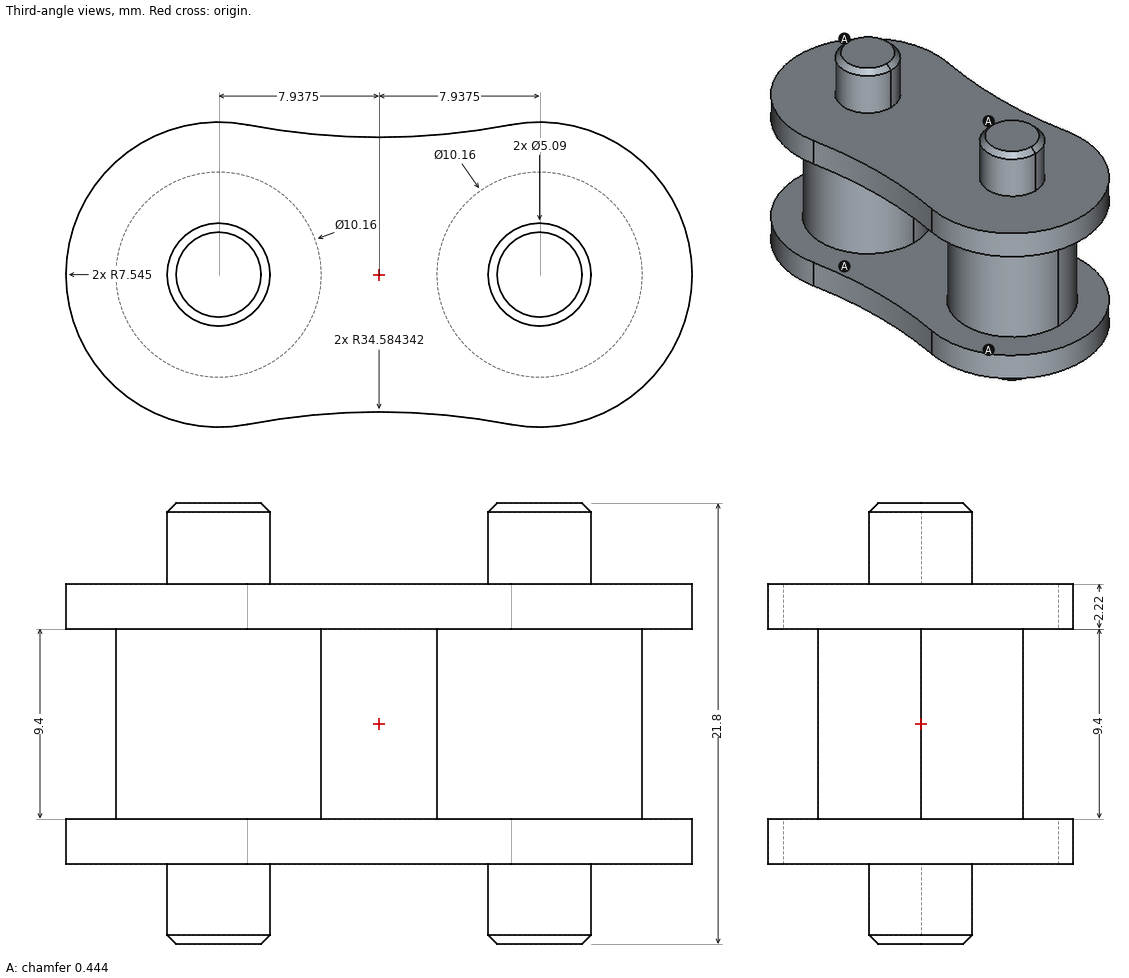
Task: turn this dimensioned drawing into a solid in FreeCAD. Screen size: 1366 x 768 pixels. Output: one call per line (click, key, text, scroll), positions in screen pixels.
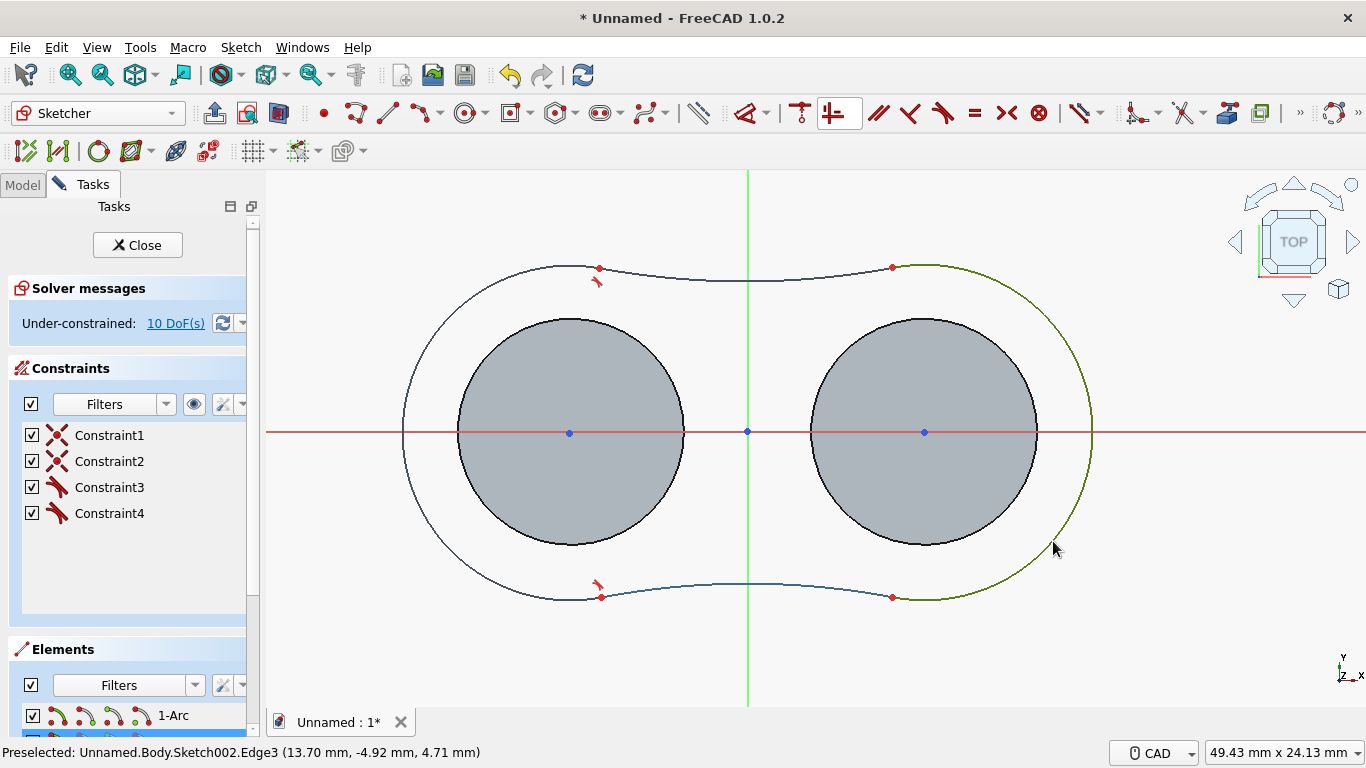
key(t)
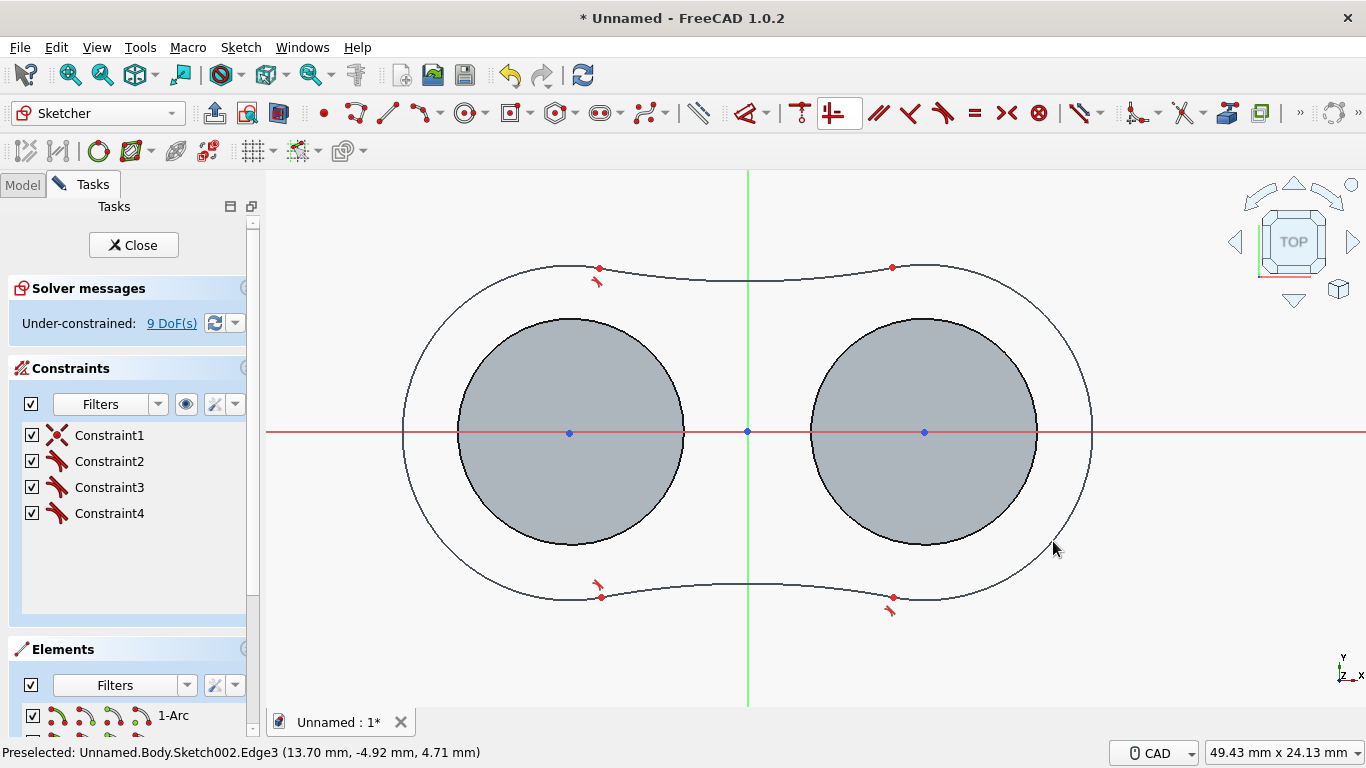
click(1053, 541)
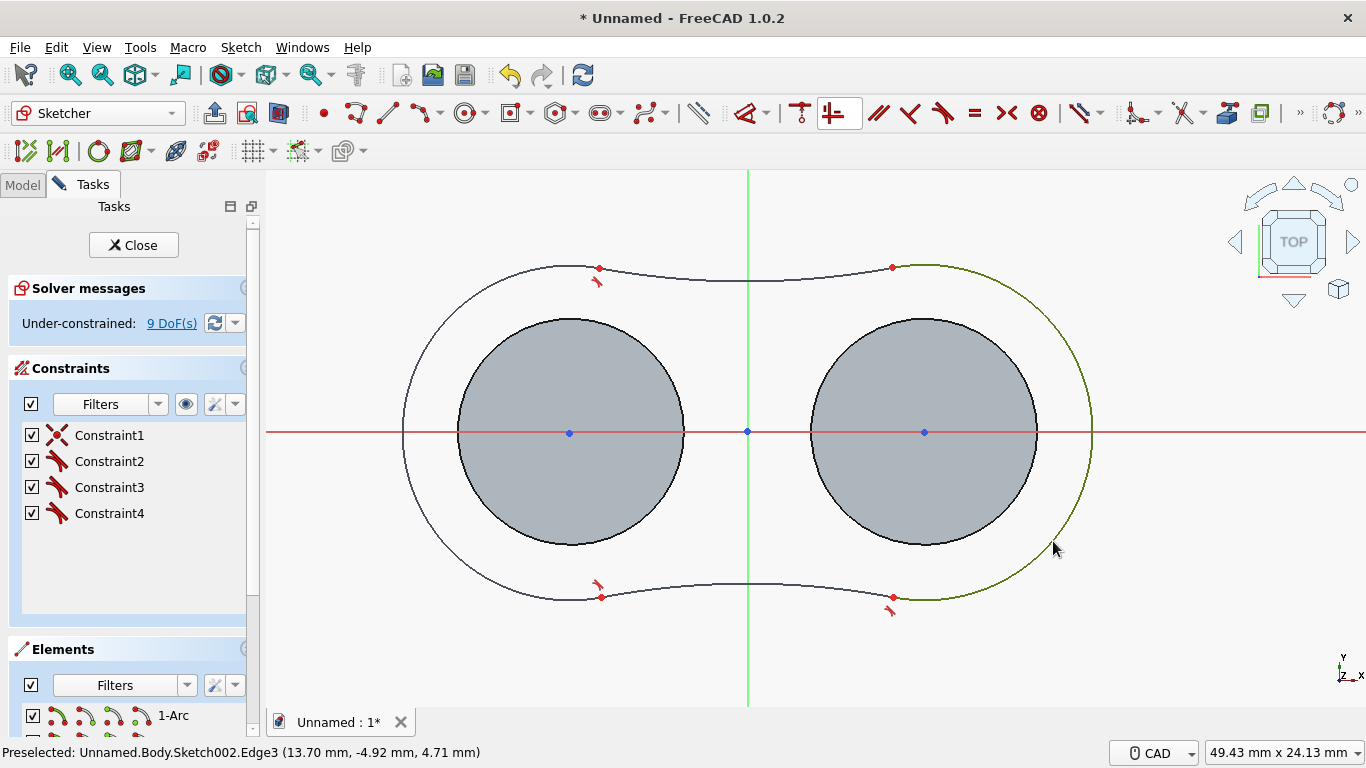
click(687, 279)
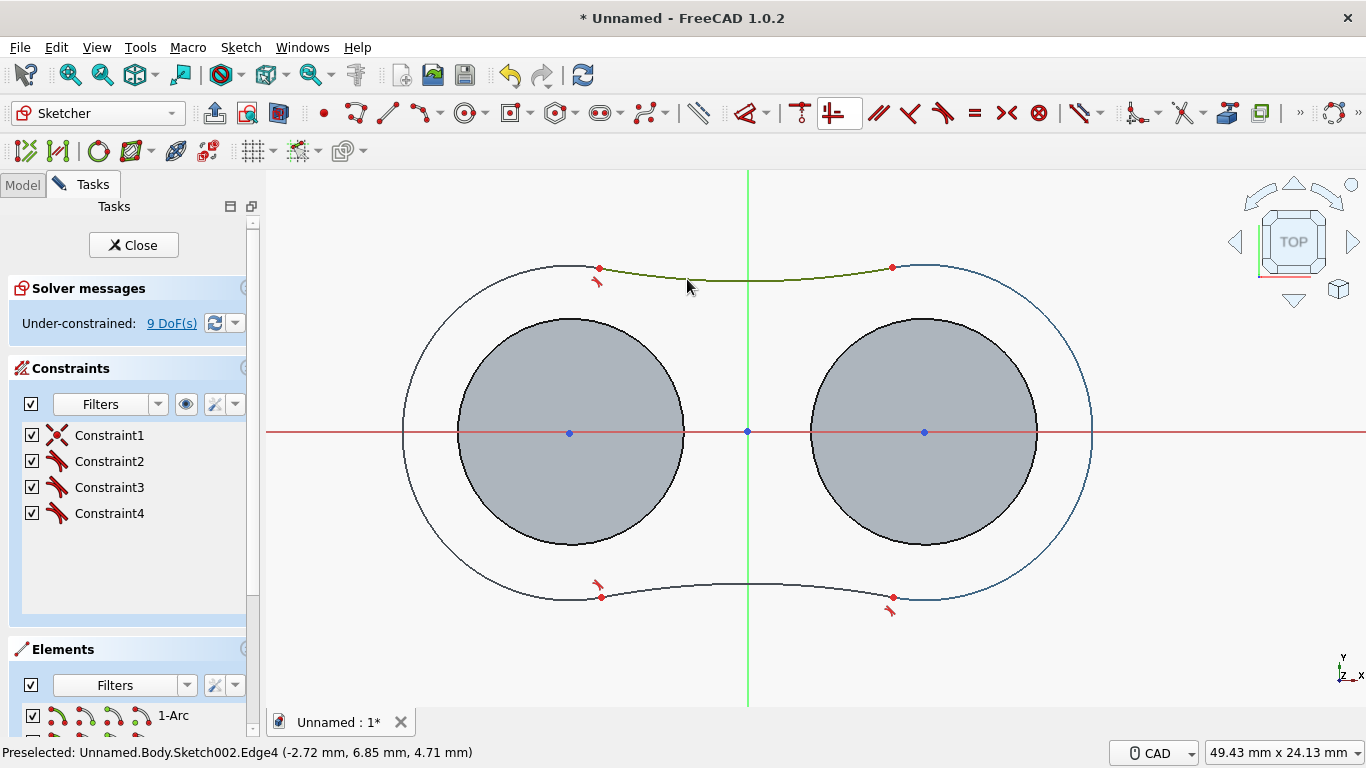
key(t)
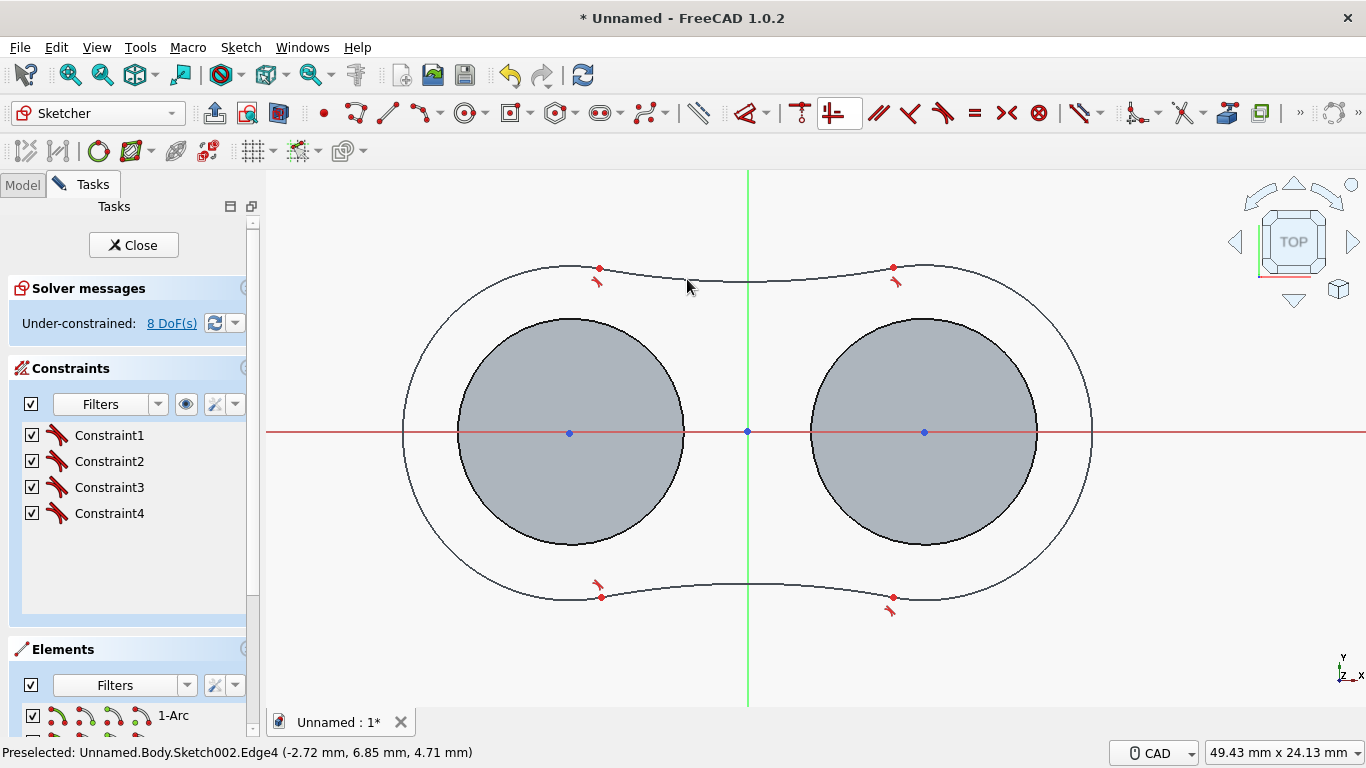
click(442, 326)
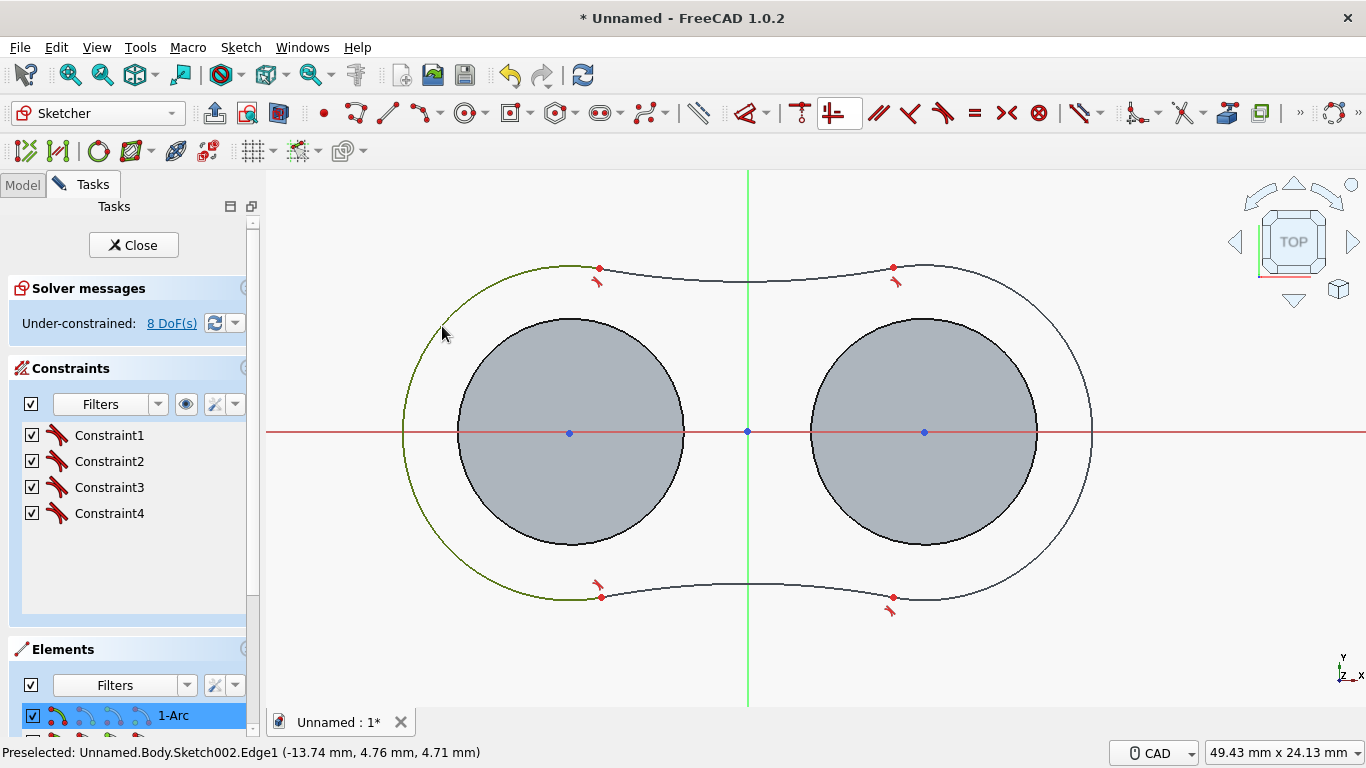
click(1052, 541)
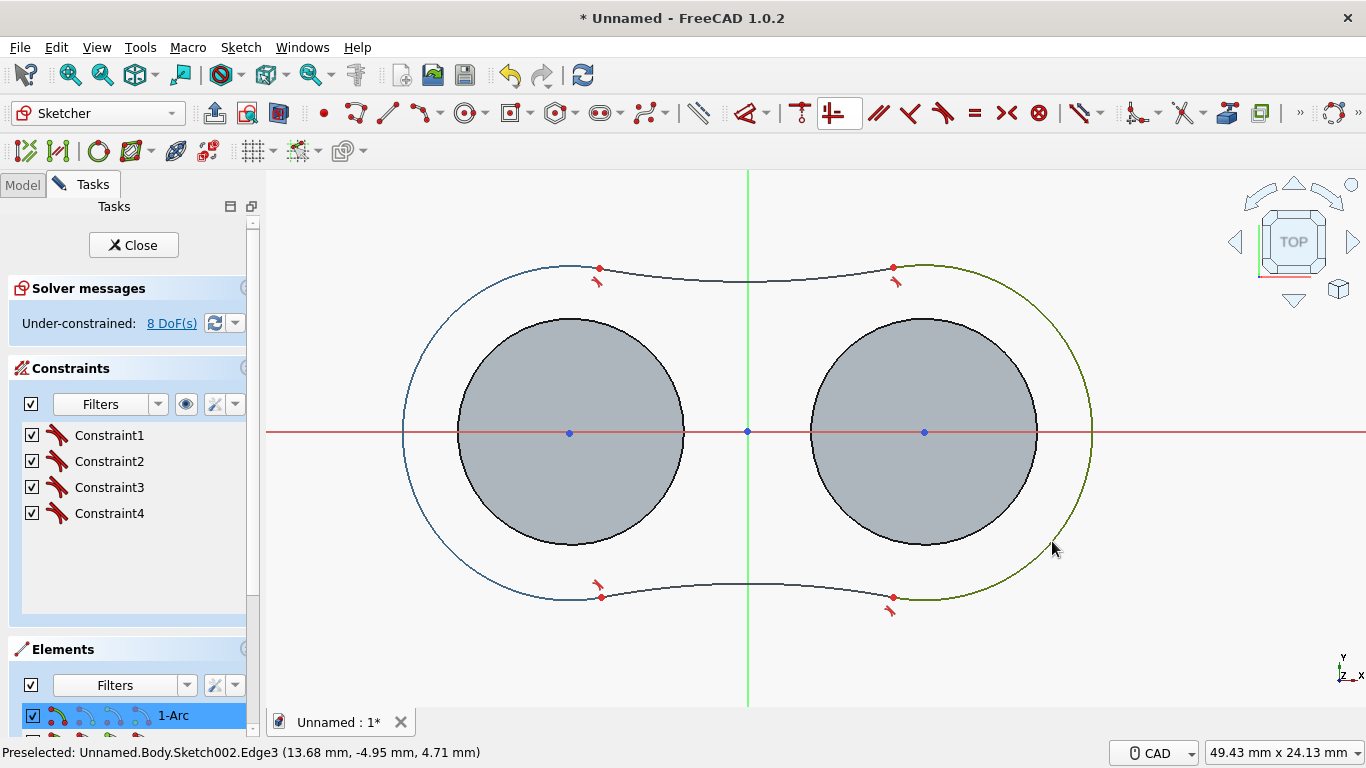
key(e)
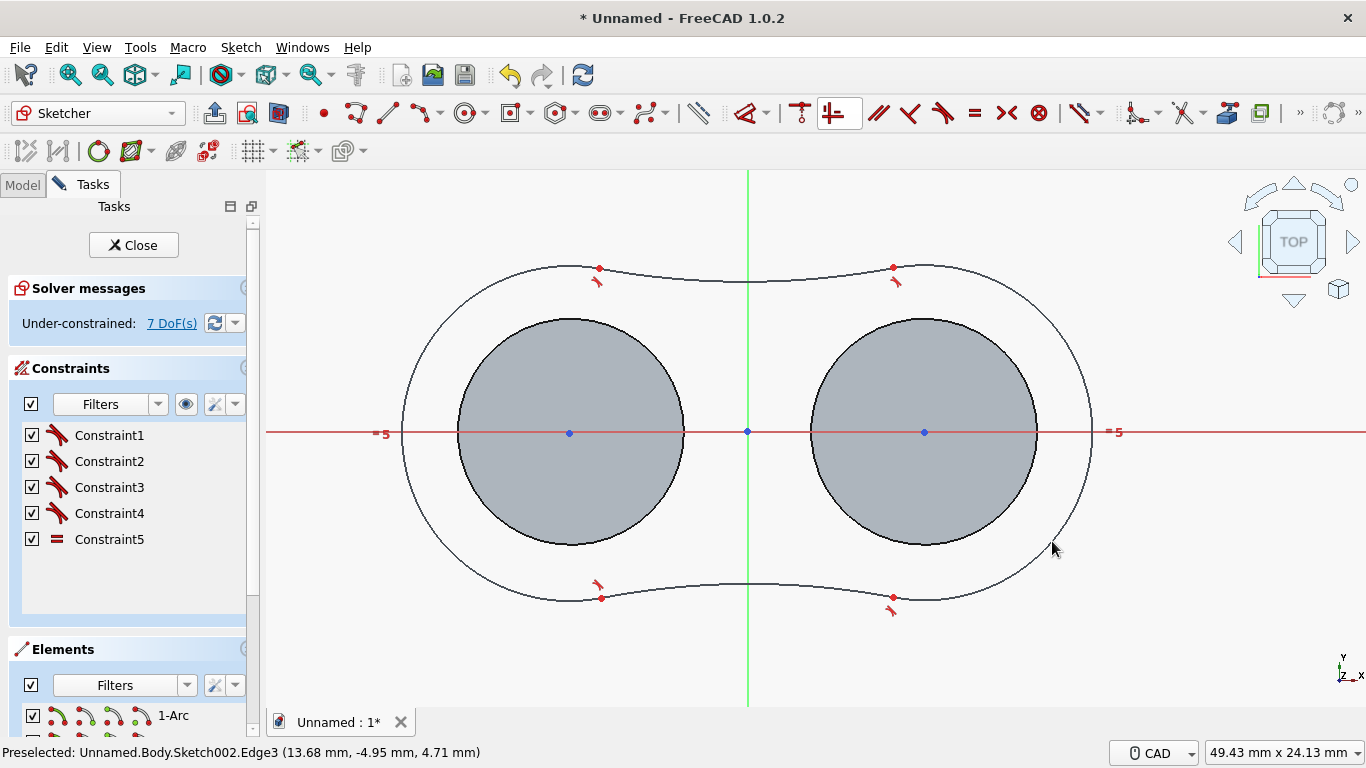
click(806, 586)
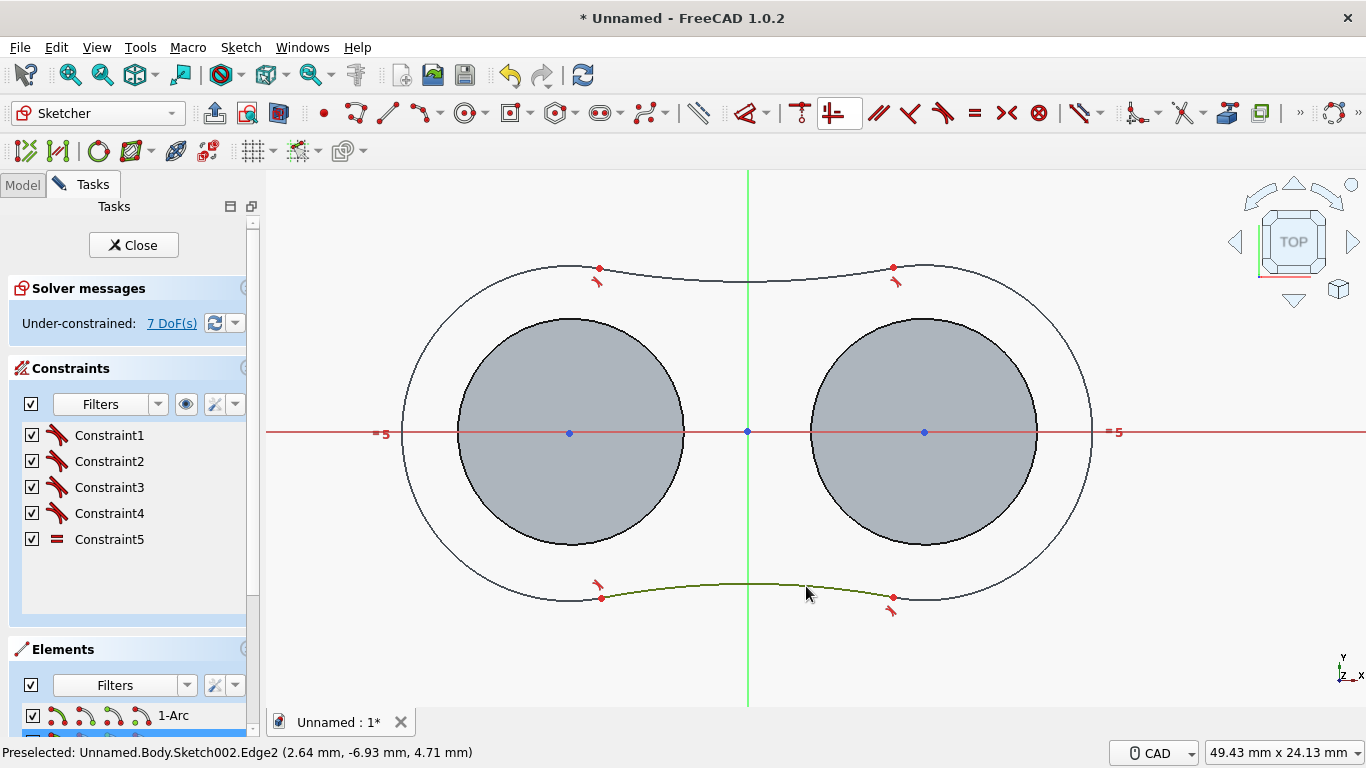
click(688, 280)